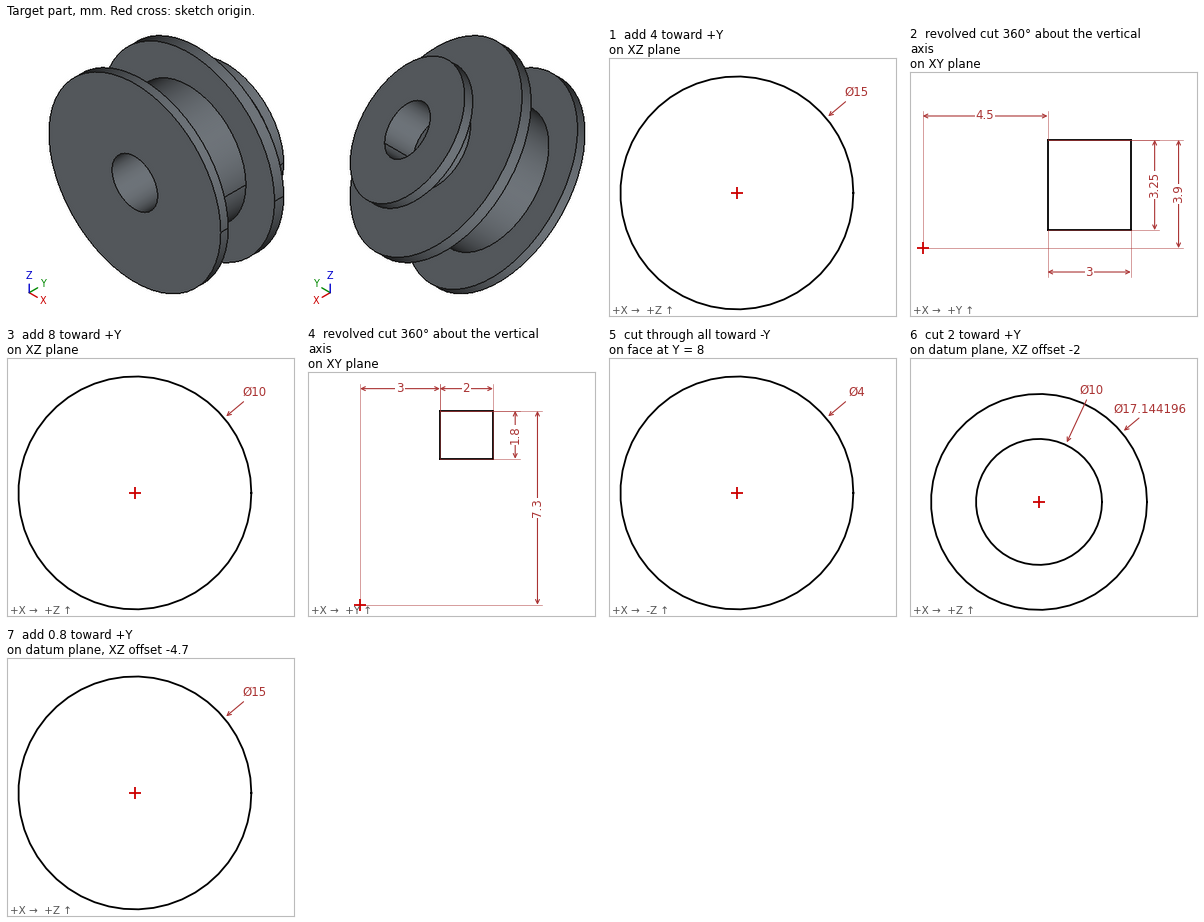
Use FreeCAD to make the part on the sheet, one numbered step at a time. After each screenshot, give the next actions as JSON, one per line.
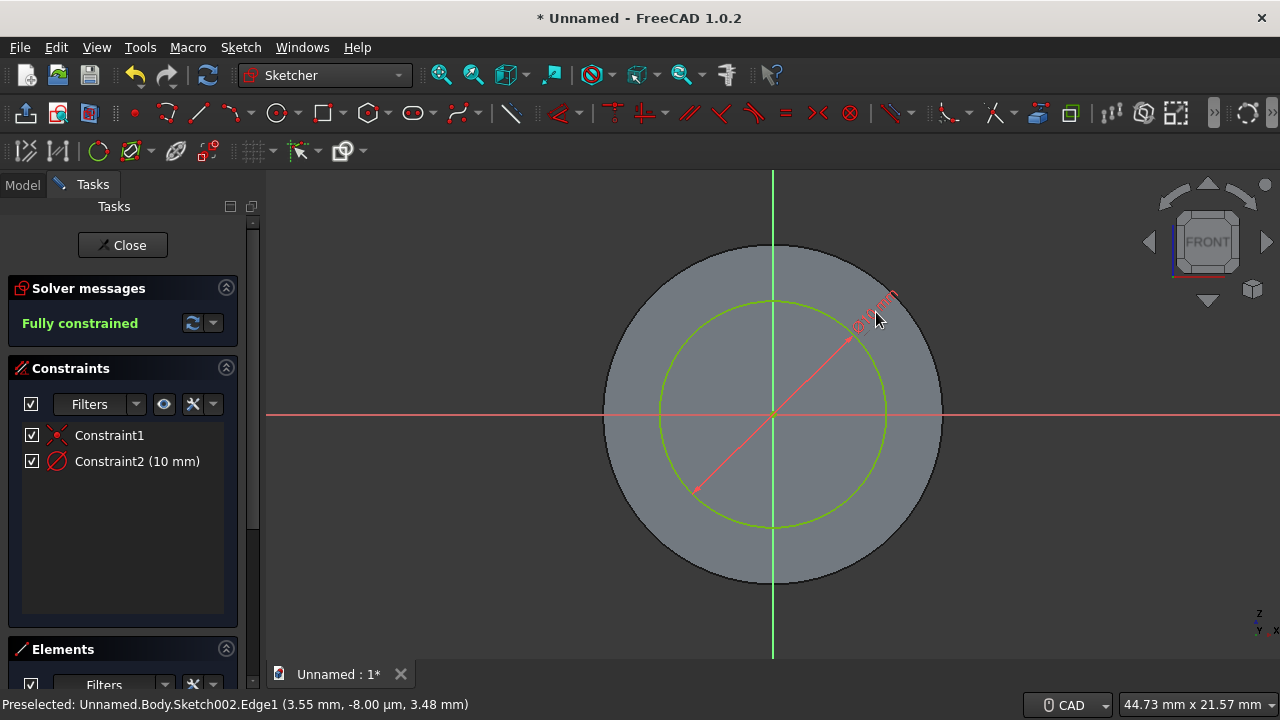
{"action": "left_click", "coordinate": [123, 245]}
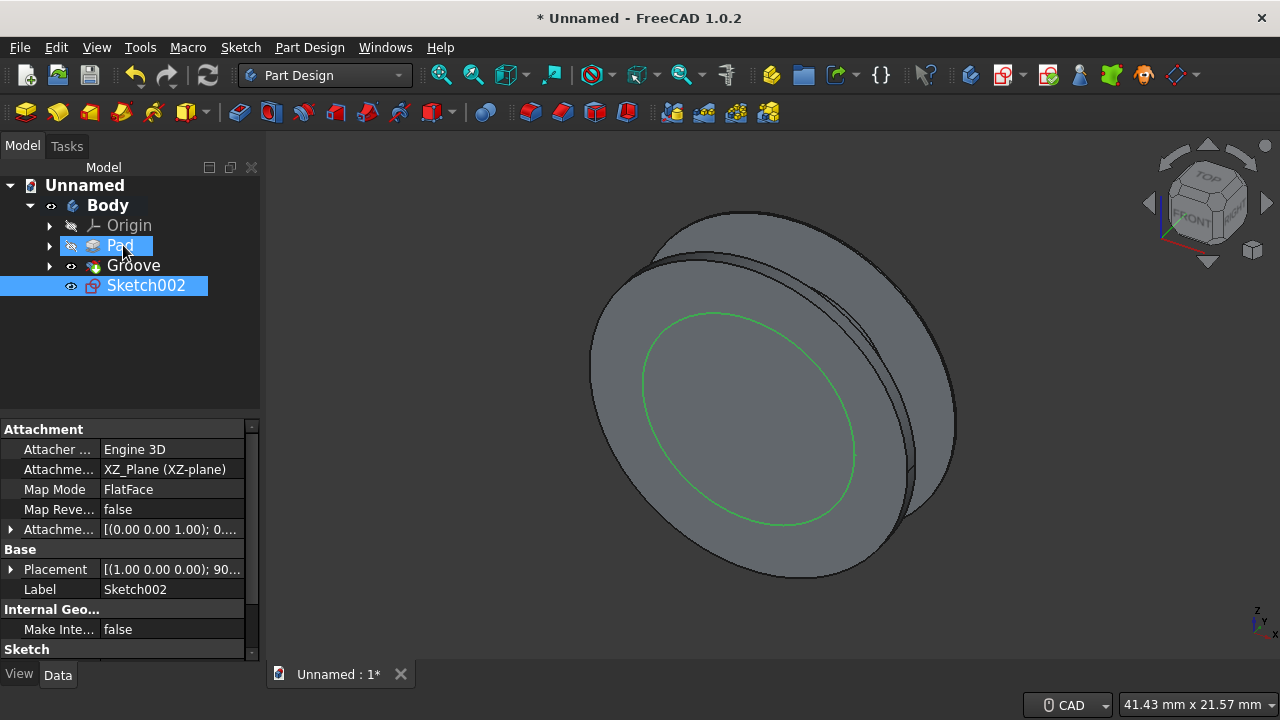
{"action": "left_click", "coordinate": [26, 112]}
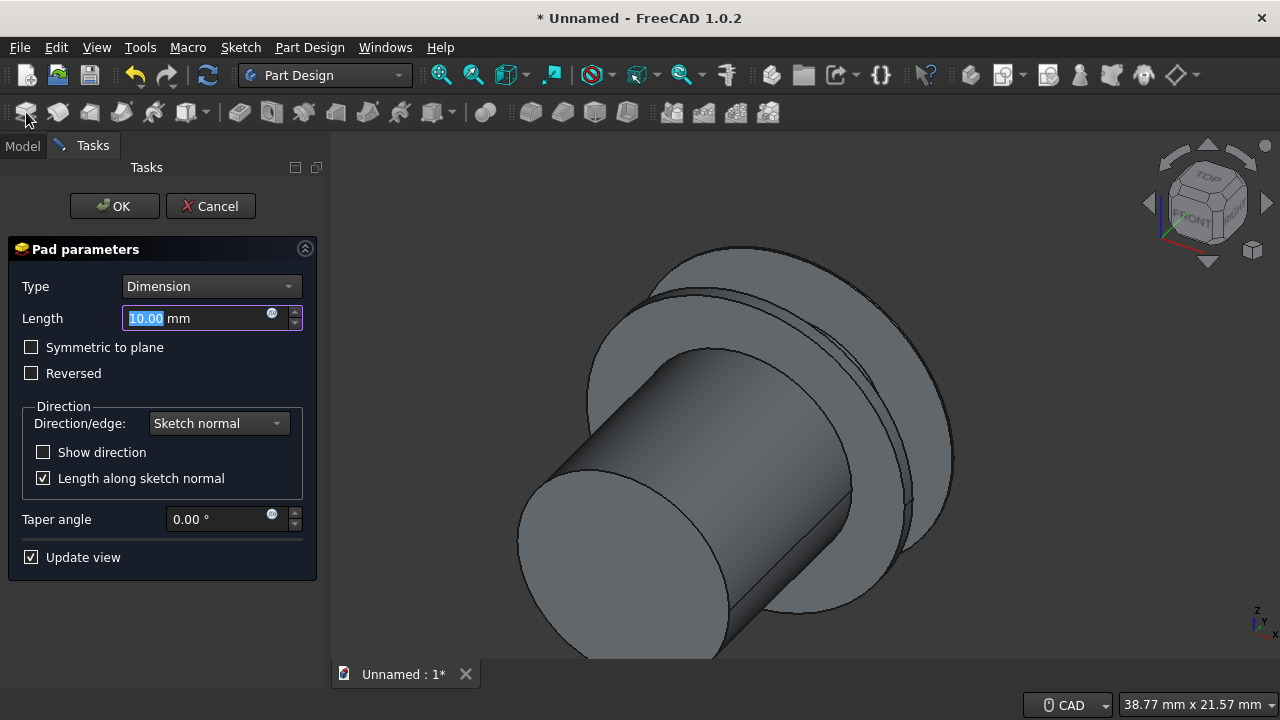
{"action": "type", "text": "8"}
{"action": "key", "text": "Tab"}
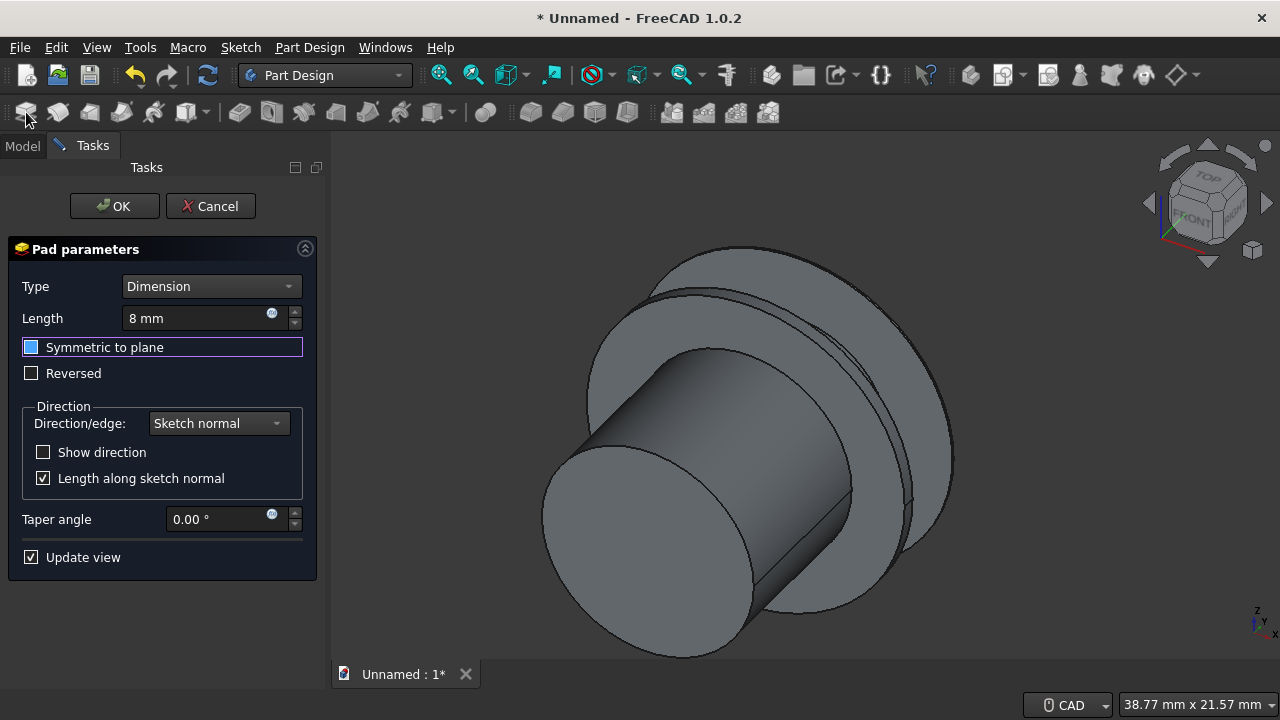
{"action": "left_click", "coordinate": [30, 373]}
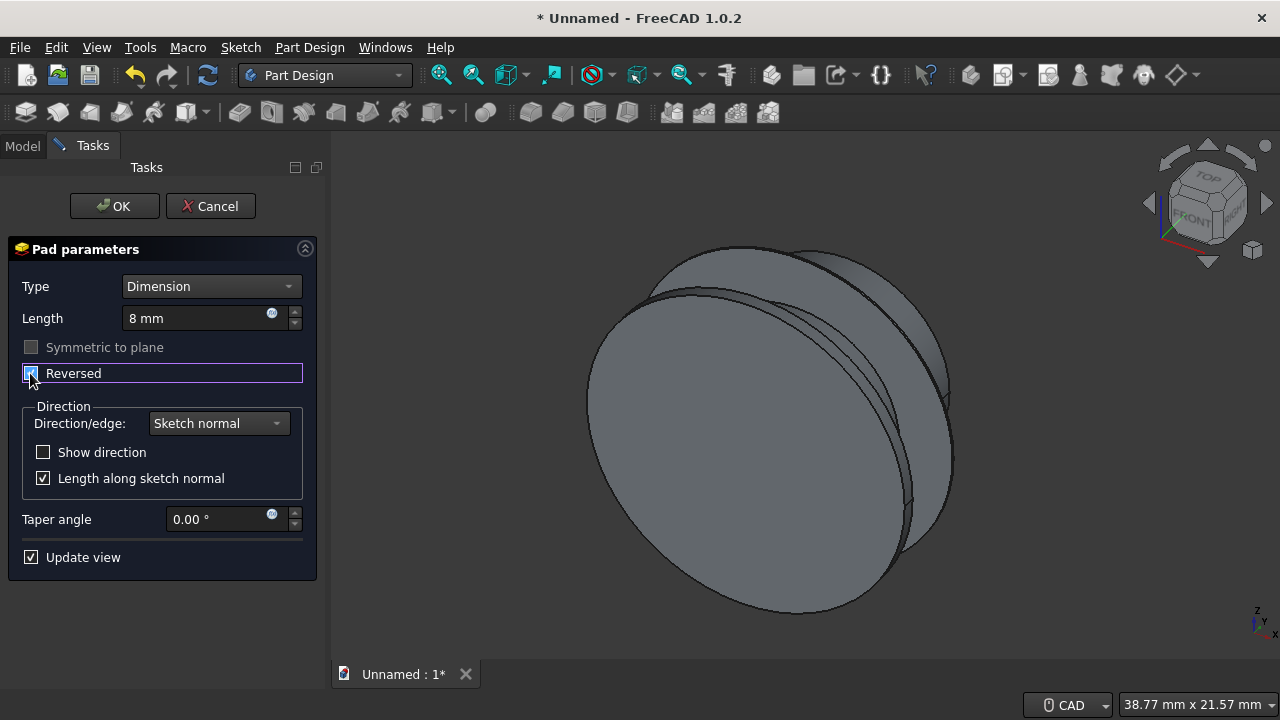
{"action": "left_click", "coordinate": [115, 206]}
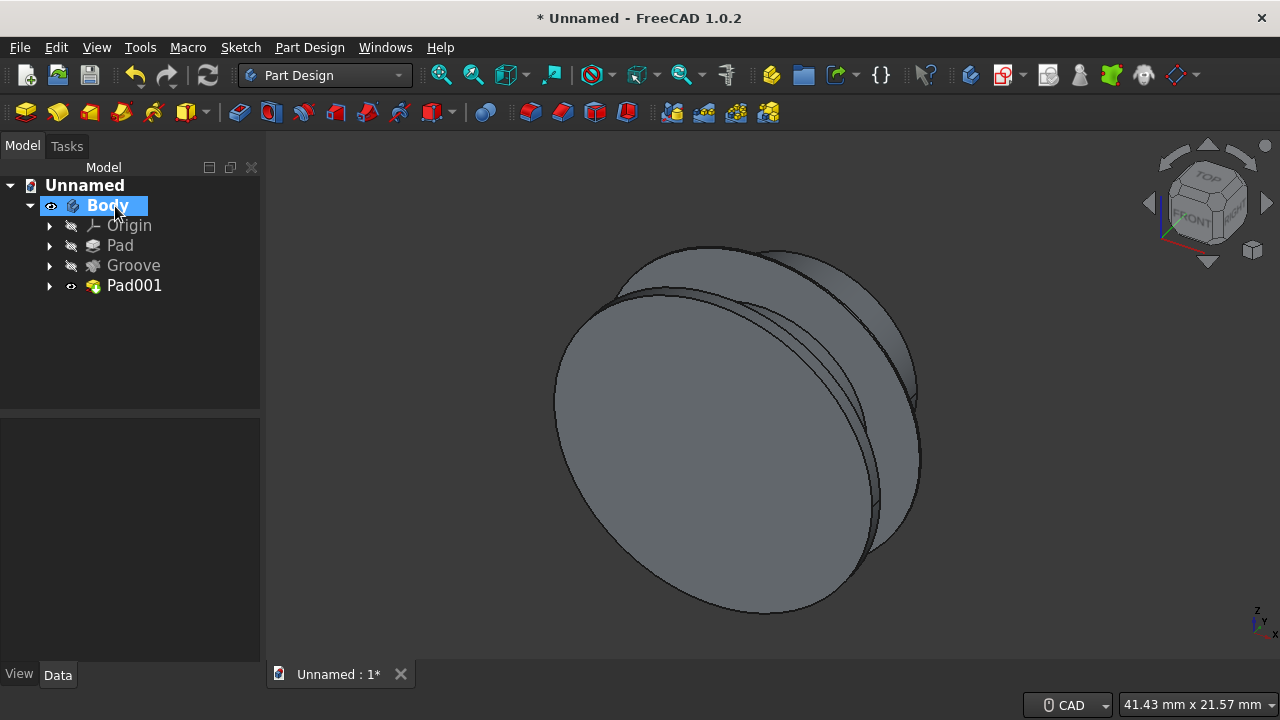
{"action": "left_click", "coordinate": [1004, 76]}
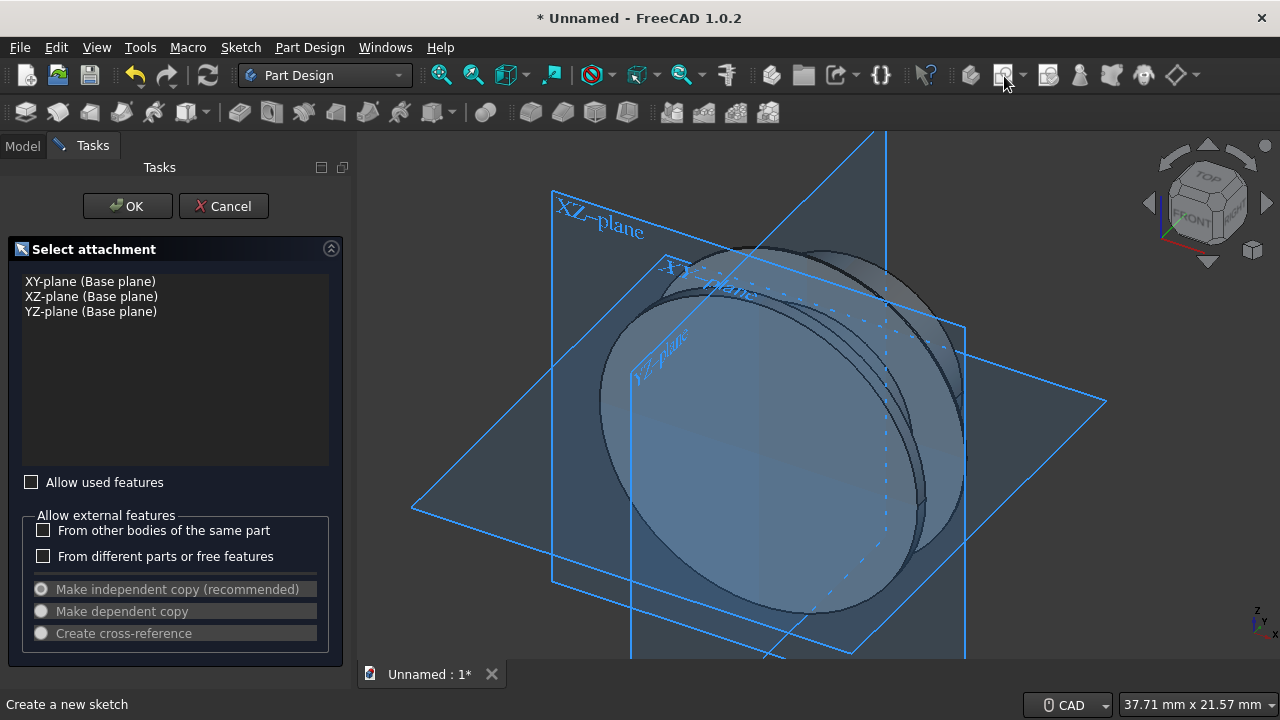
{"action": "left_click", "coordinate": [82, 282]}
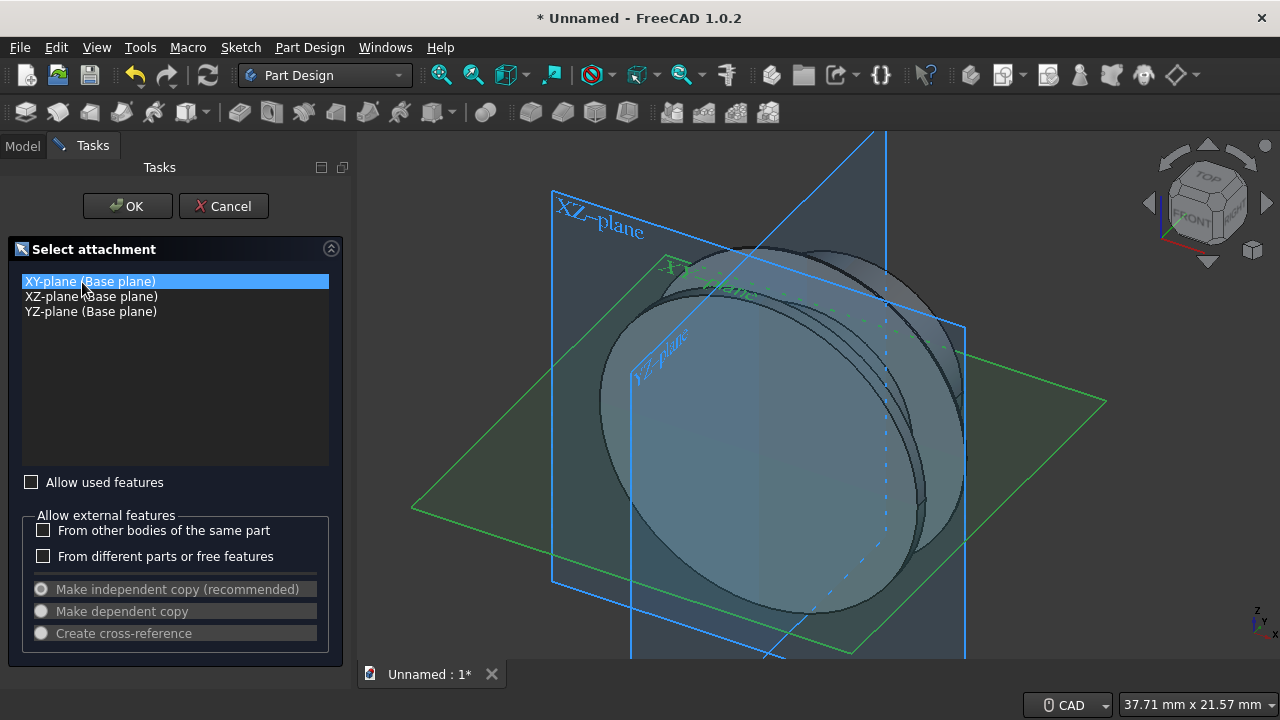
{"action": "left_click", "coordinate": [128, 206]}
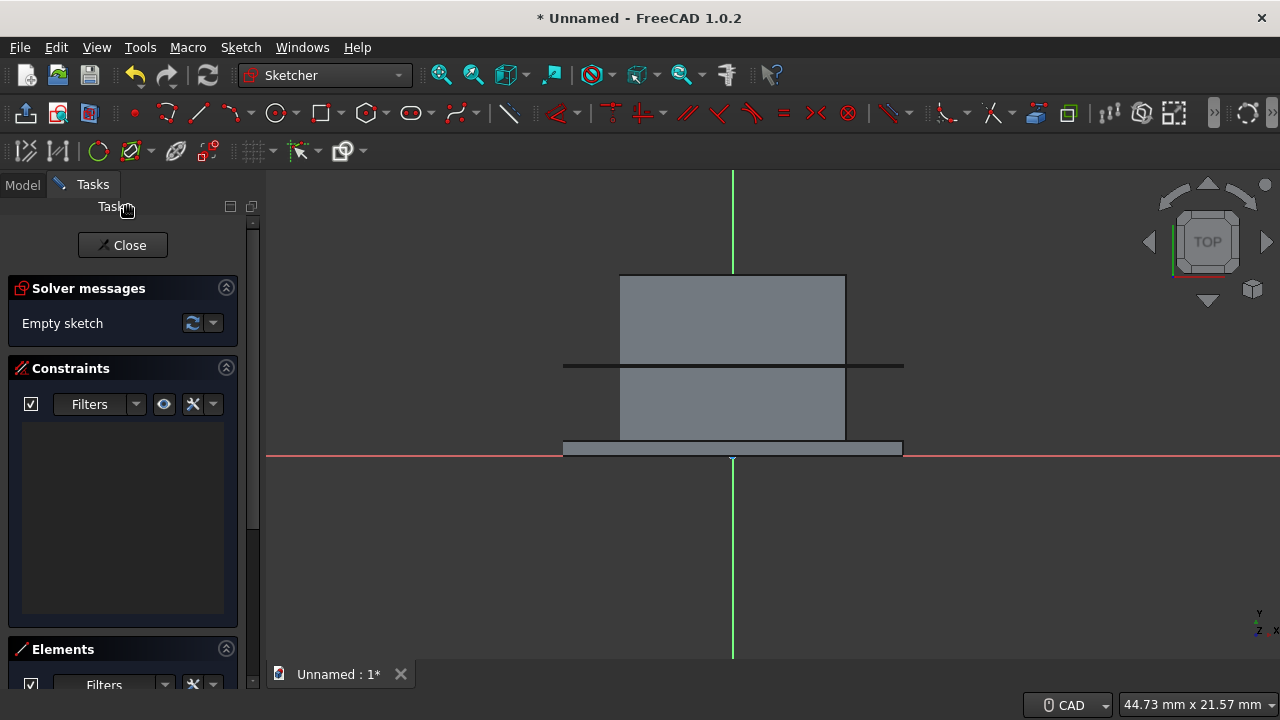
{"action": "key", "text": "q s"}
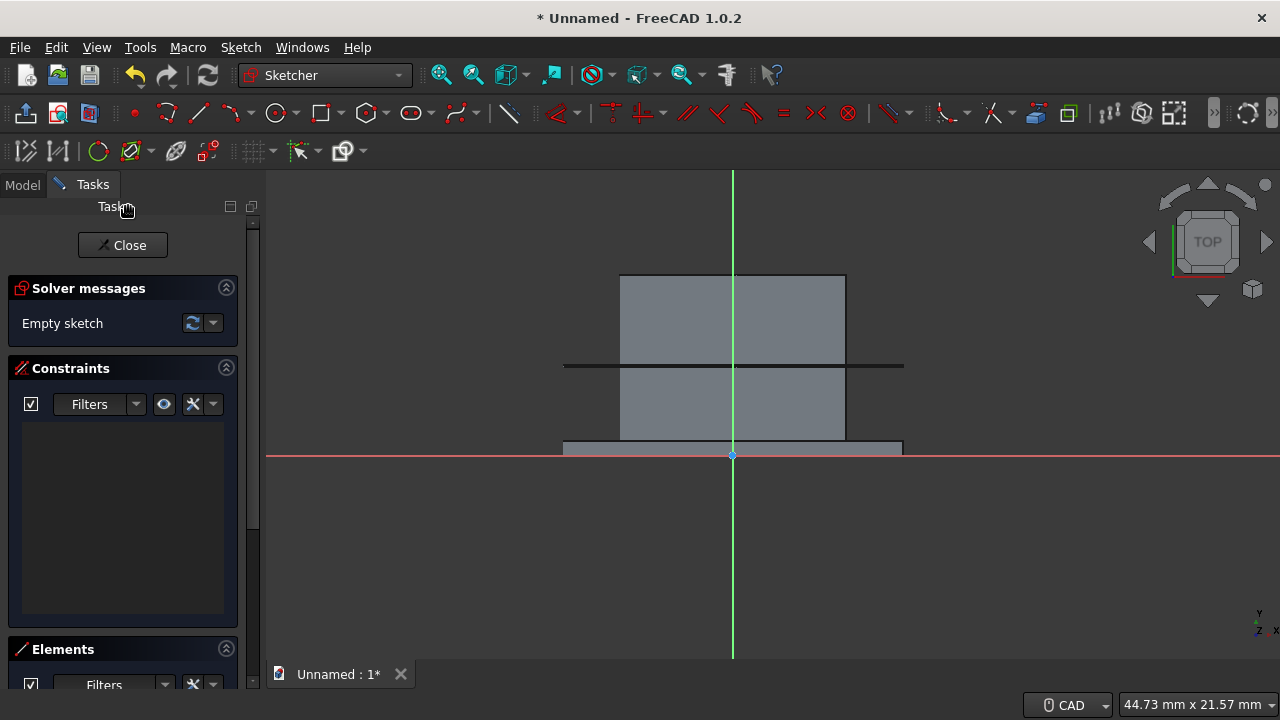
{"action": "scroll", "coordinate": [842, 295], "scroll_direction": "up", "scroll_amount": 10}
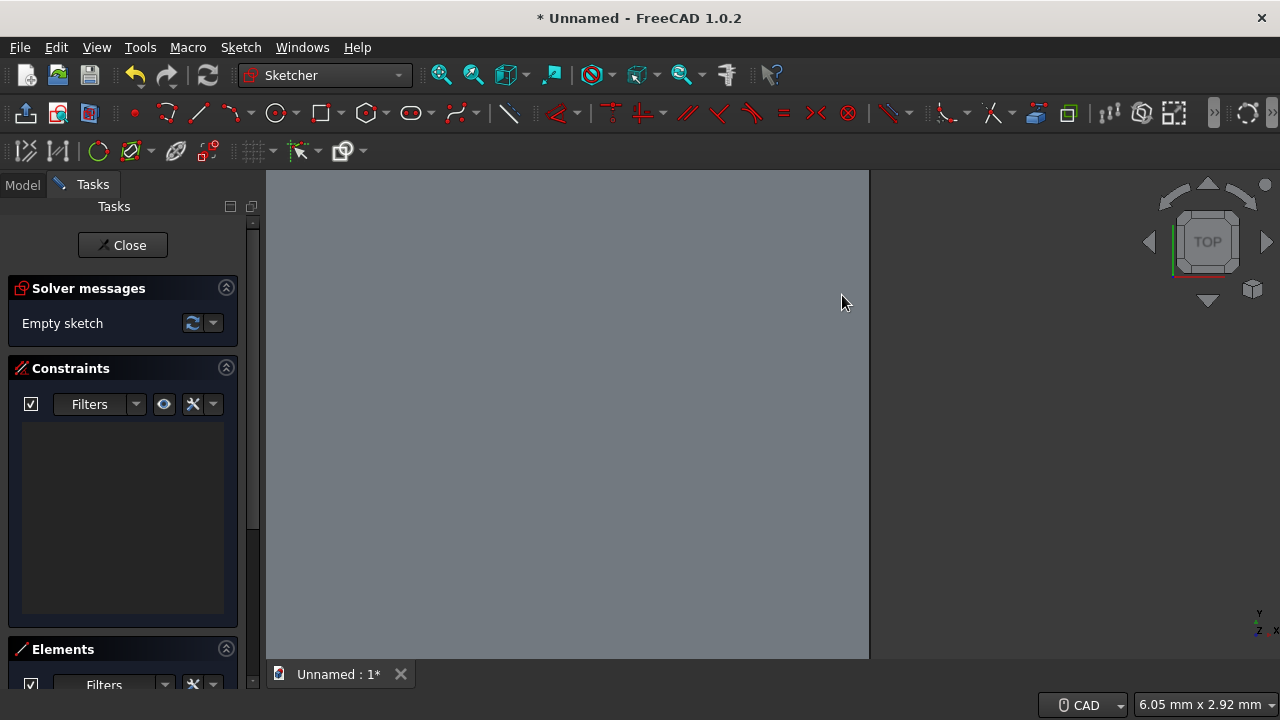
{"action": "left_click", "coordinate": [322, 114]}